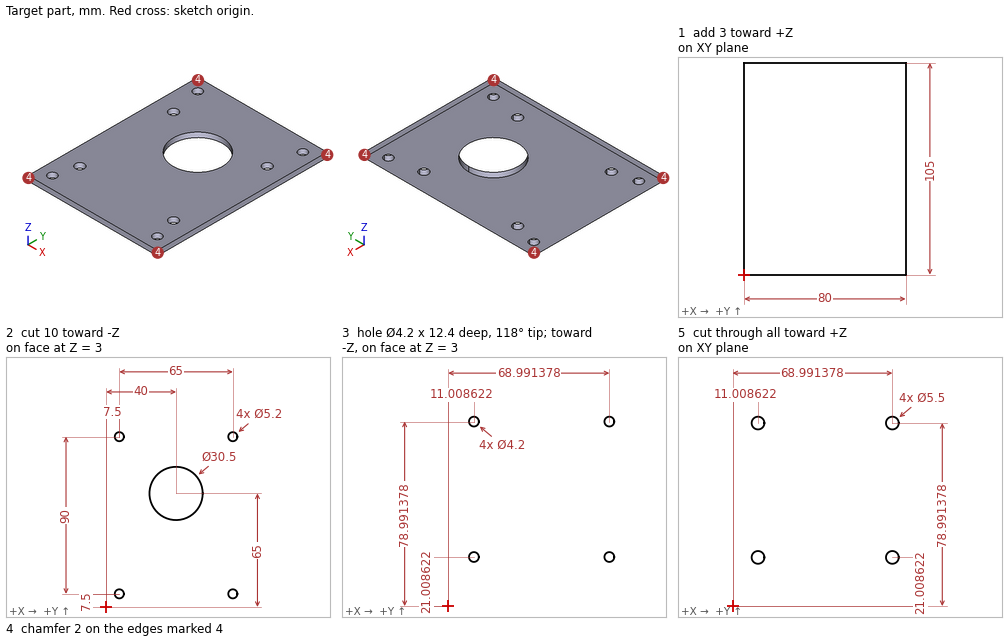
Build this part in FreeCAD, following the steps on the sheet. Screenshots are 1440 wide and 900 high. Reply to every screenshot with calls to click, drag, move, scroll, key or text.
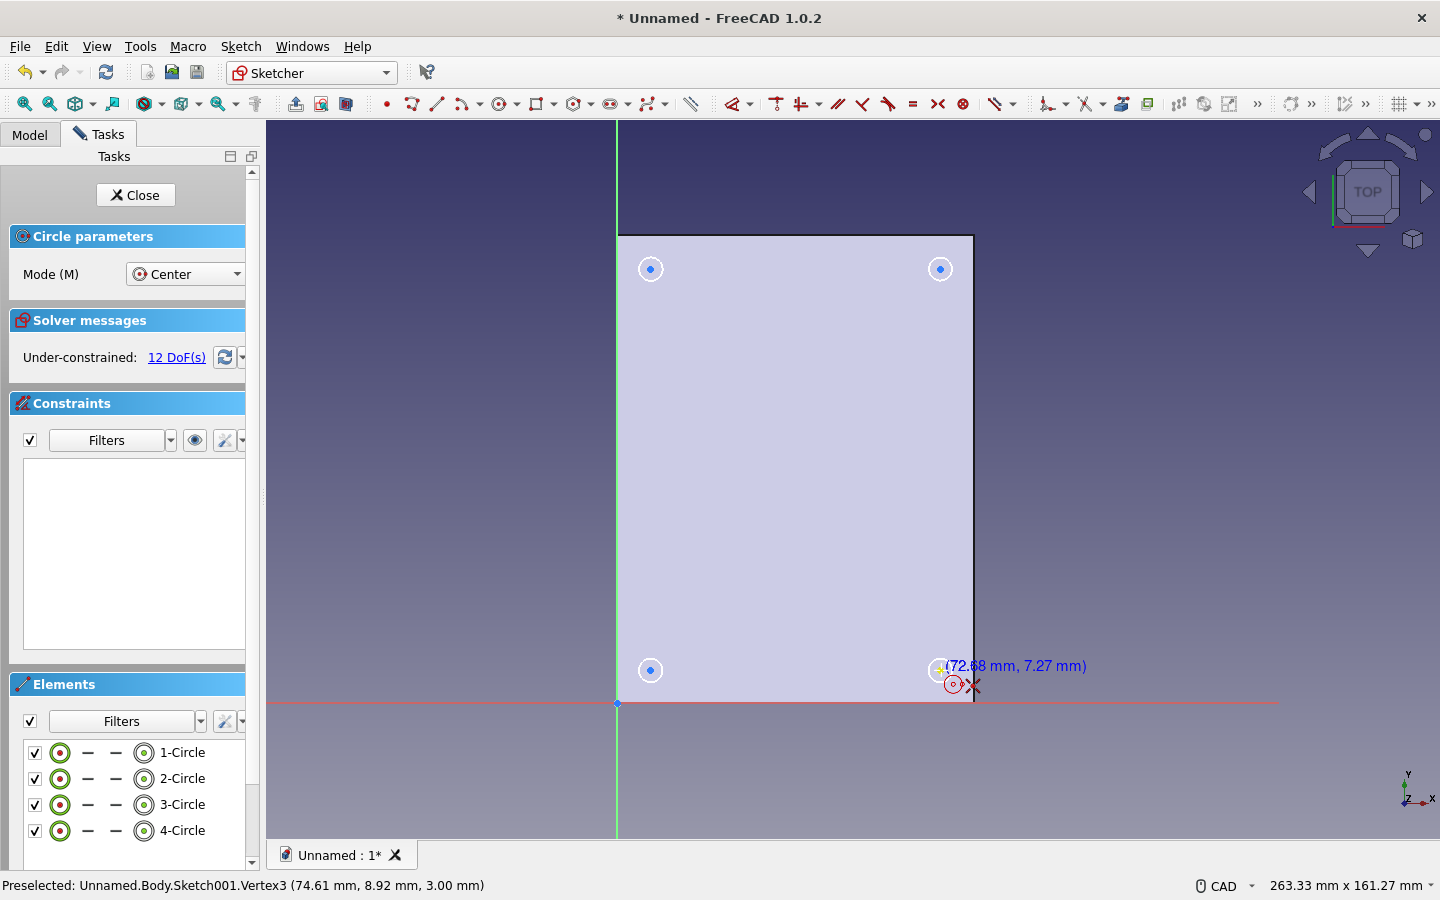
click(796, 413)
click(844, 365)
key(Escape)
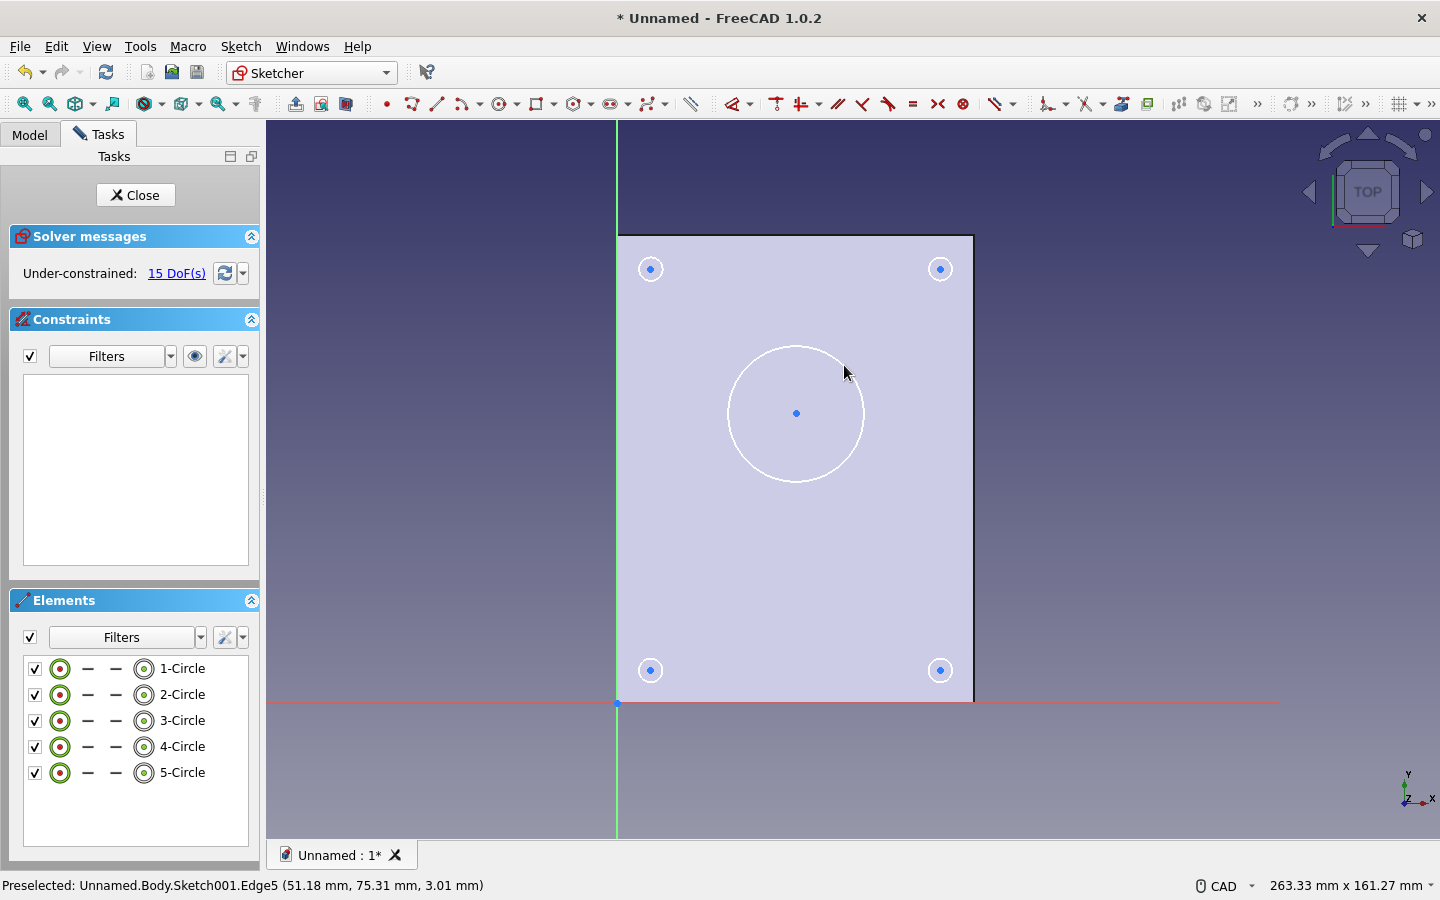
click(659, 261)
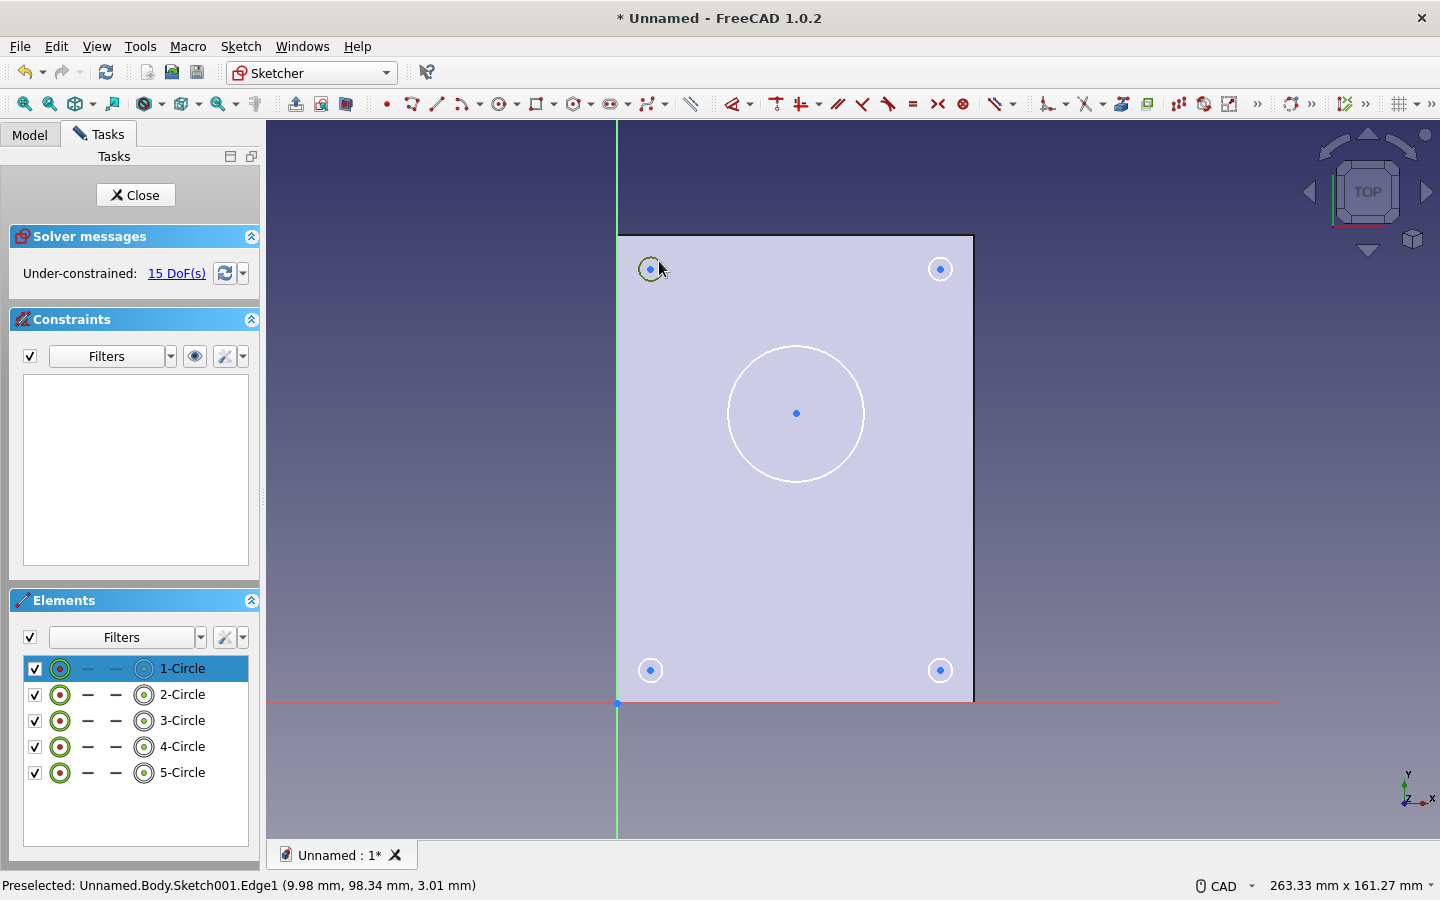
click(948, 261)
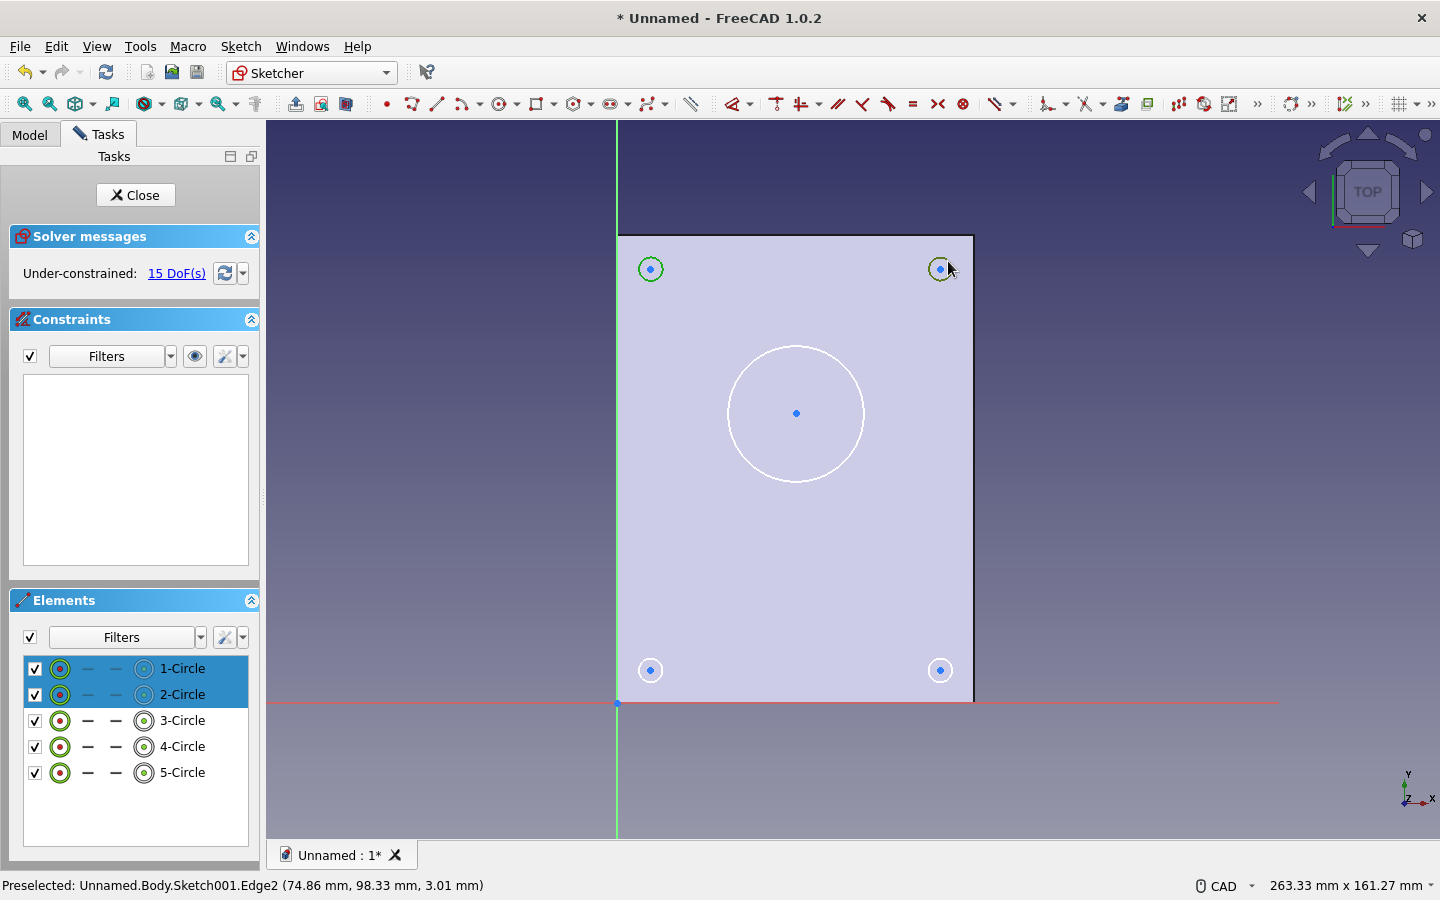
click(659, 662)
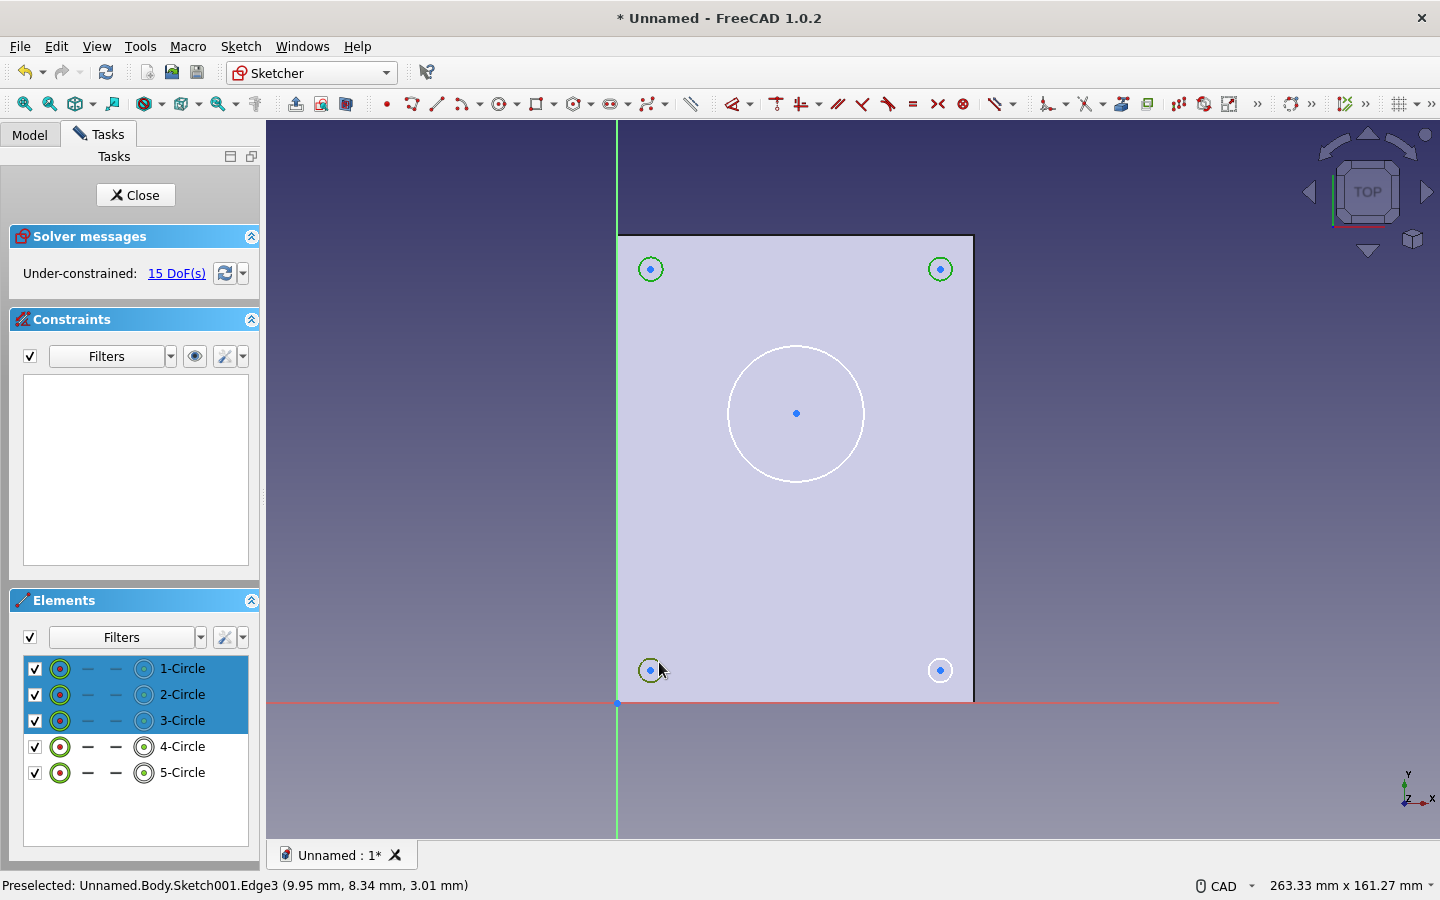
click(949, 662)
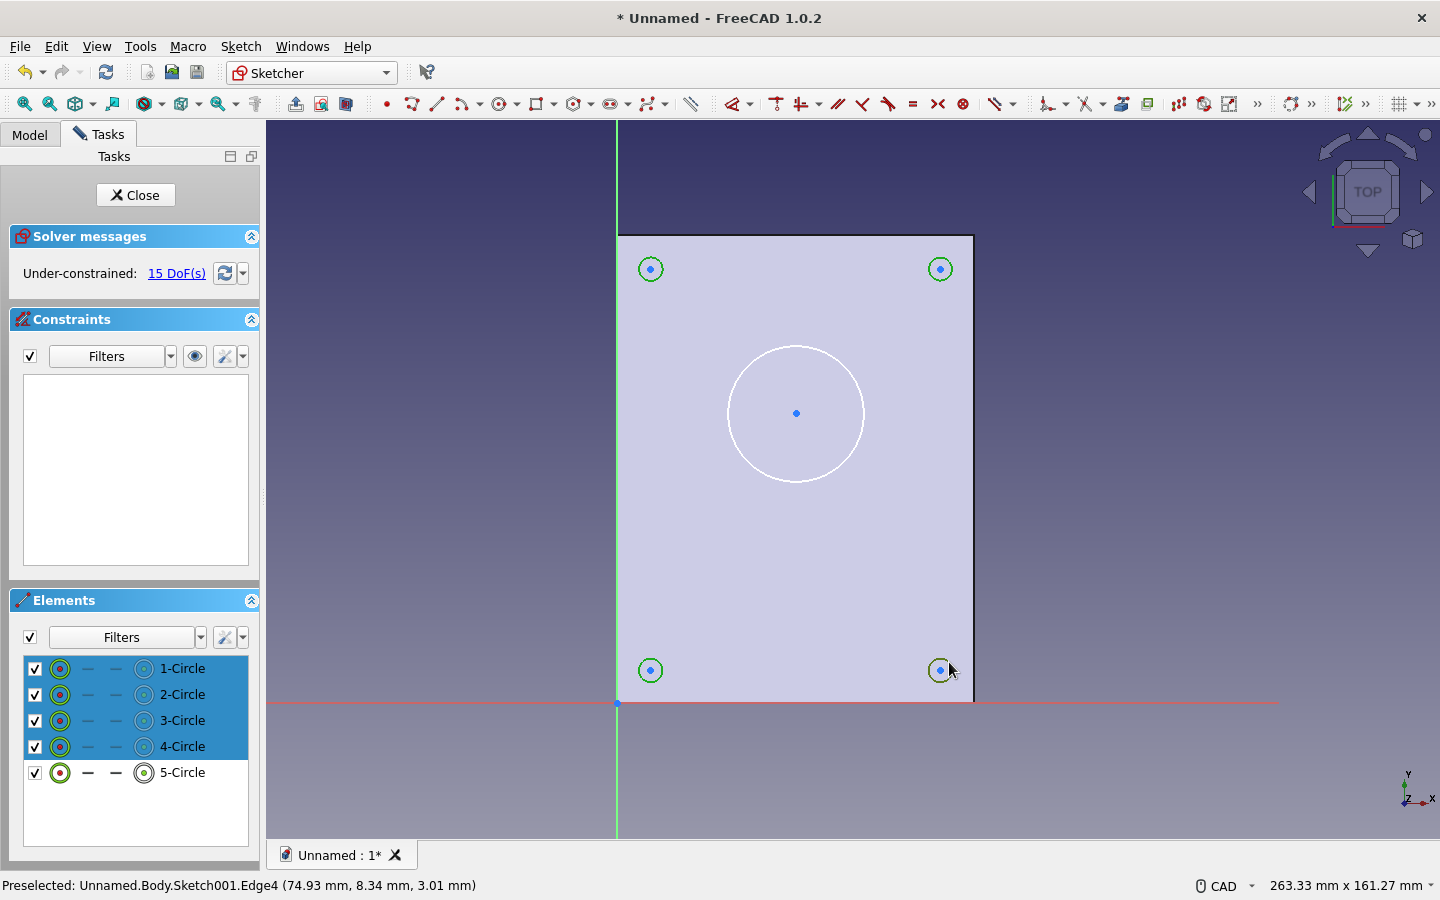
click(913, 104)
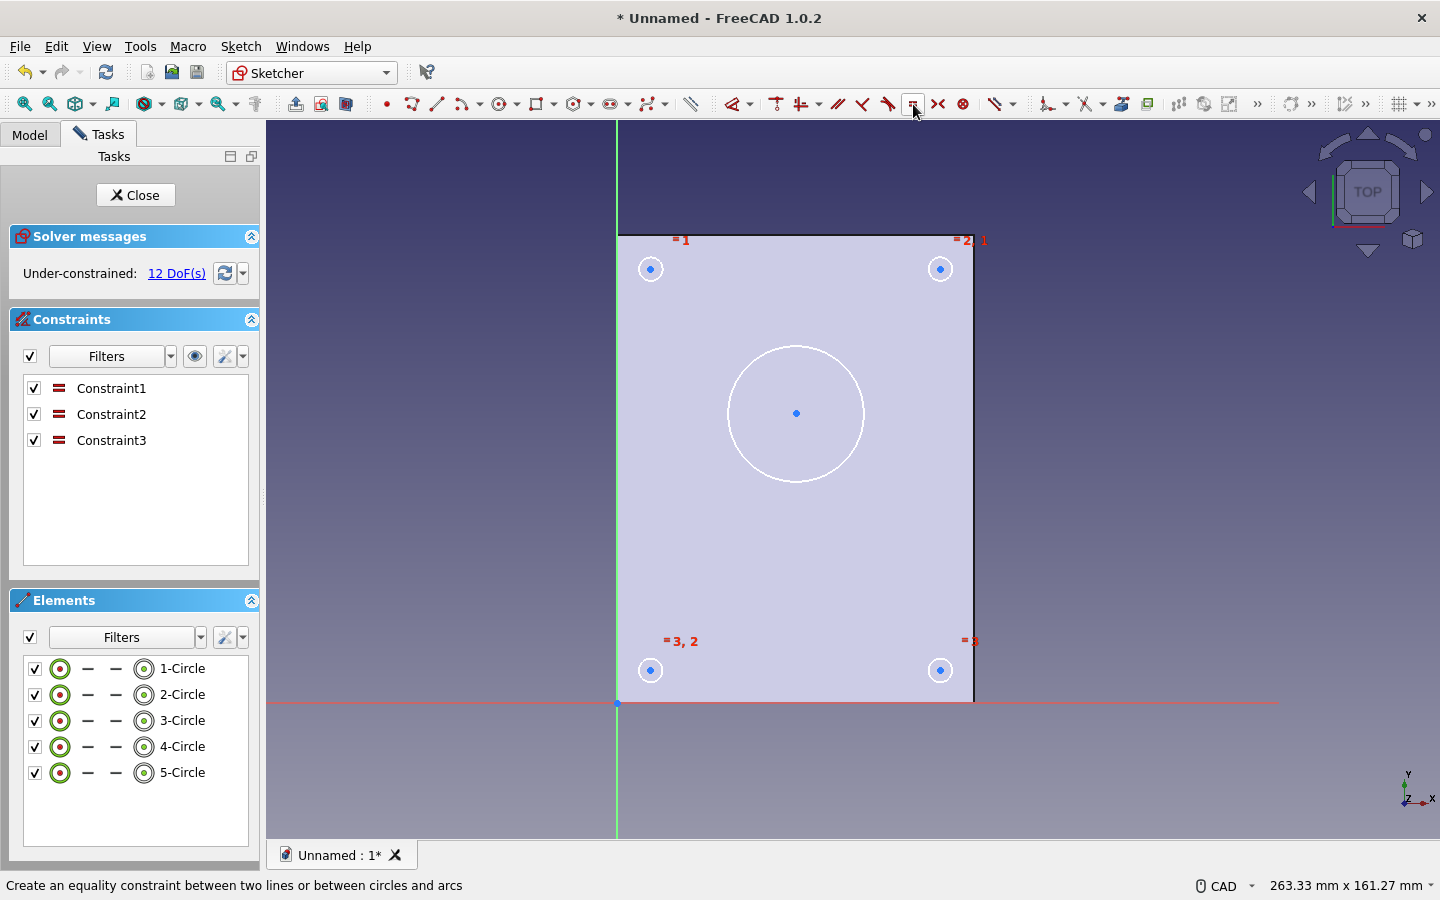
click(651, 269)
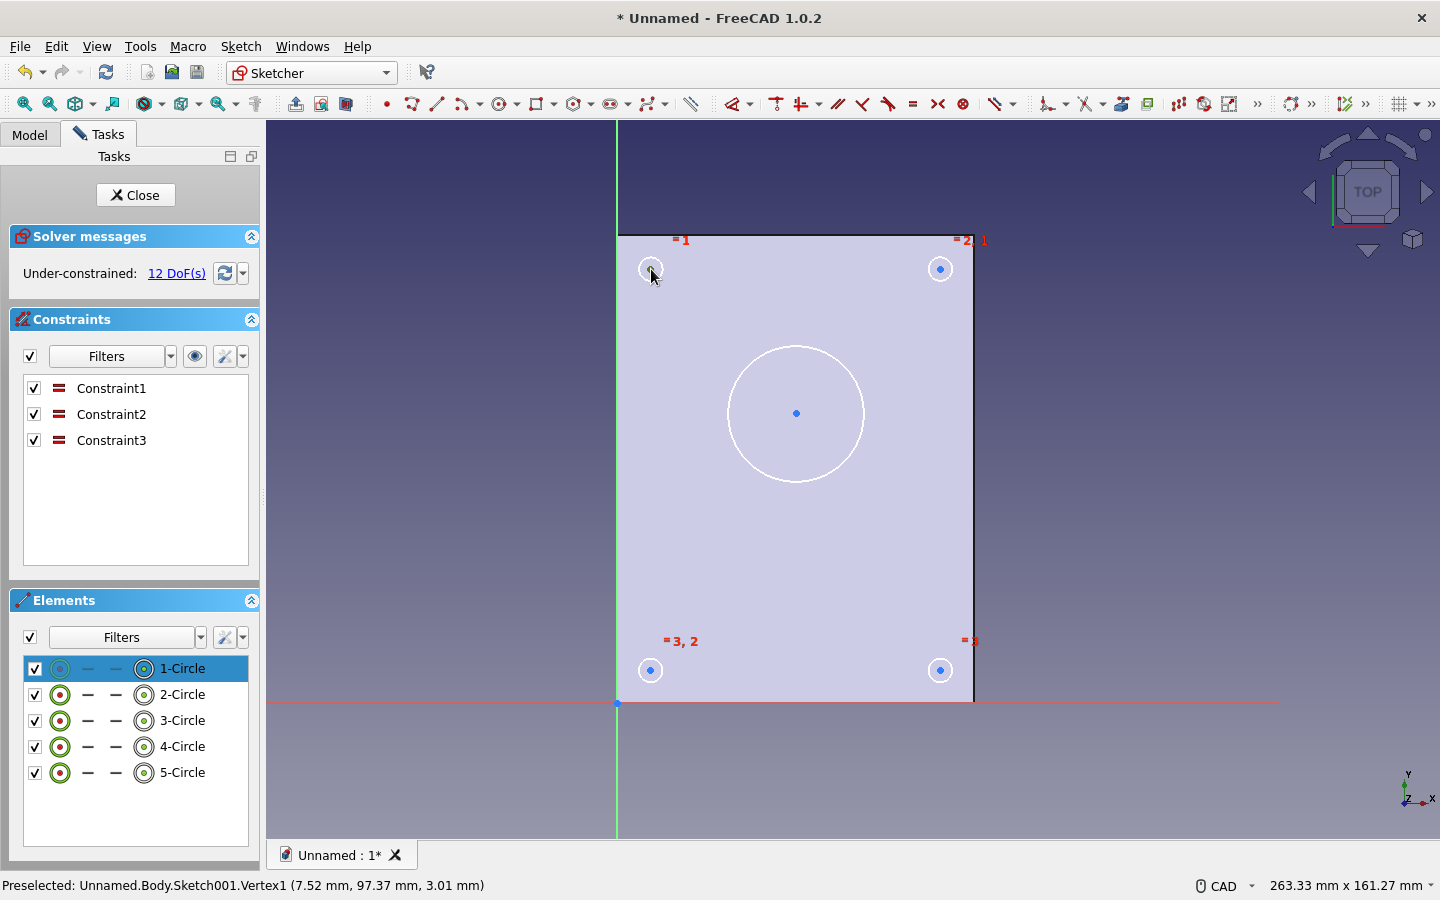
click(940, 269)